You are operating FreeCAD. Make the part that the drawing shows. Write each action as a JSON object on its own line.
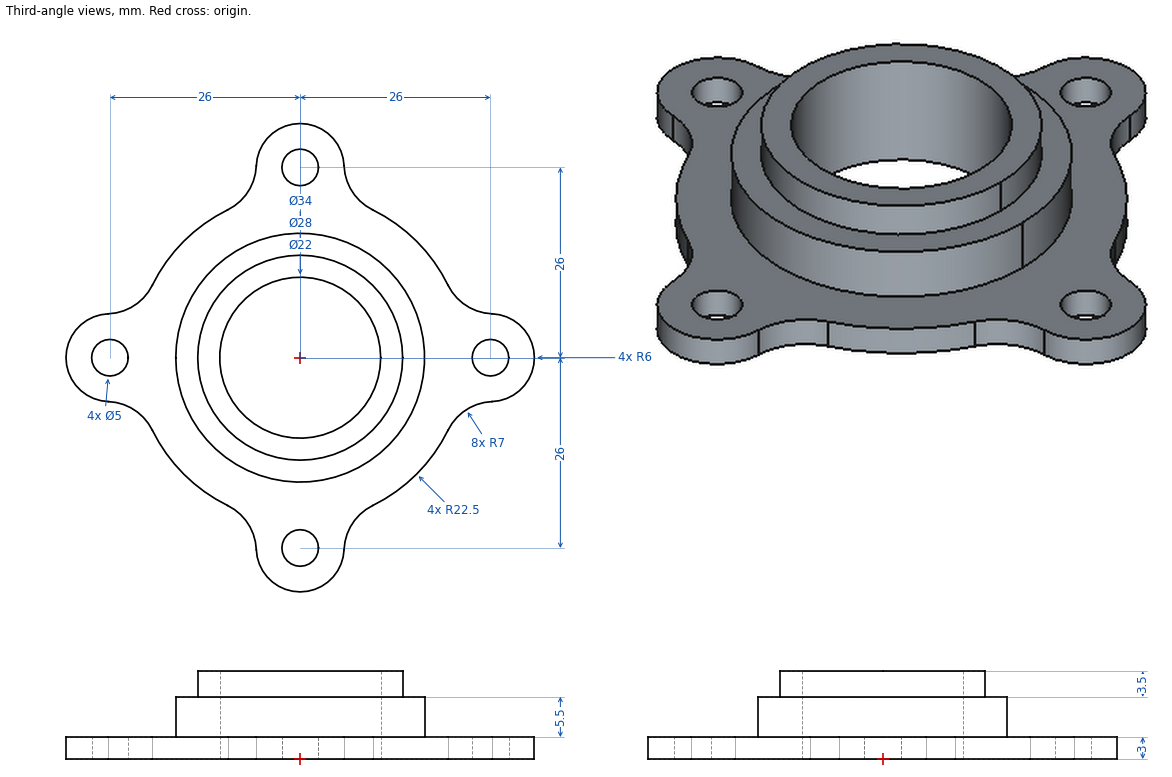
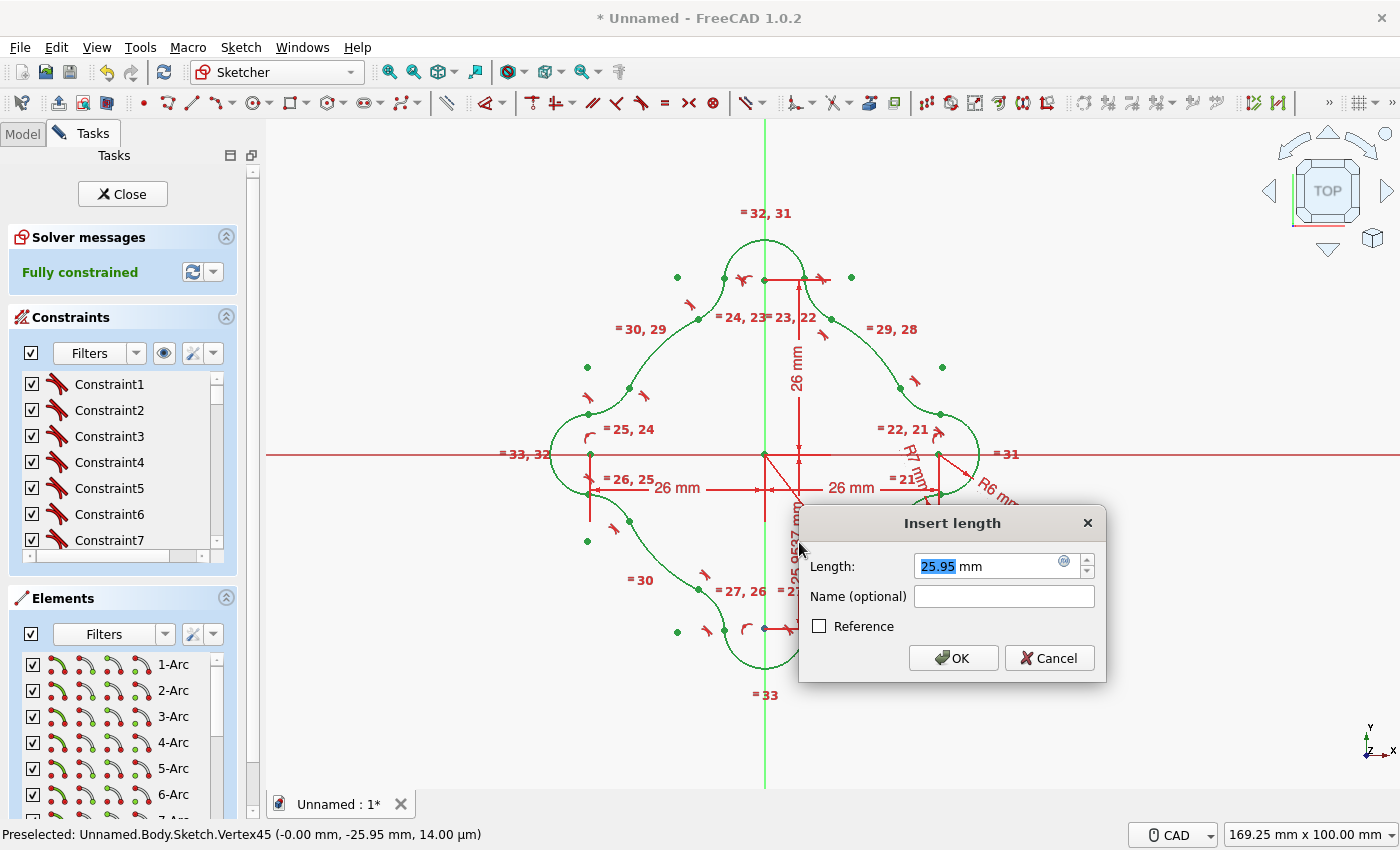
{"action": "type", "text": "26"}
{"action": "key", "text": "Return"}
{"action": "key", "text": "Escape"}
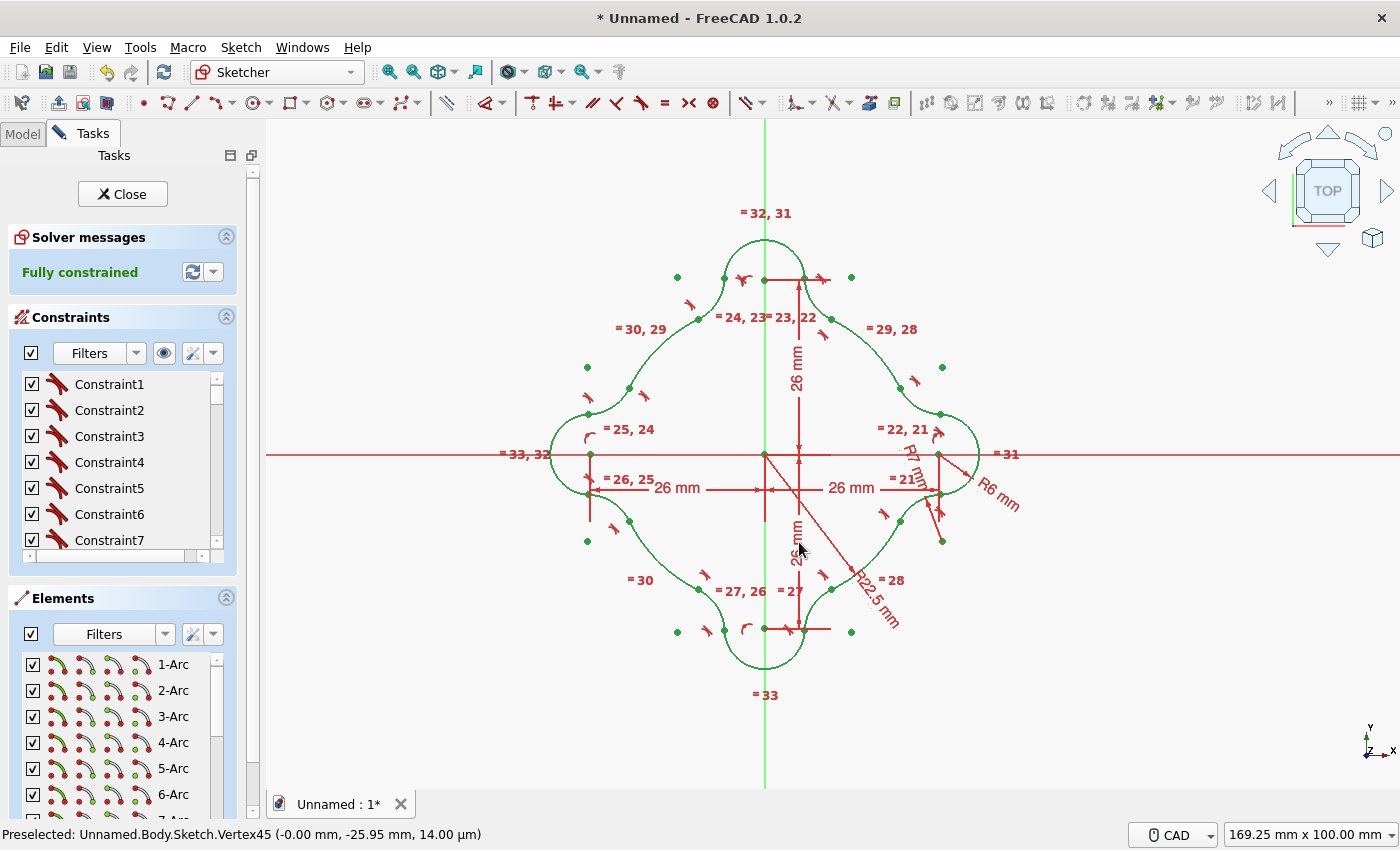
{"action": "left_click", "coordinate": [123, 194]}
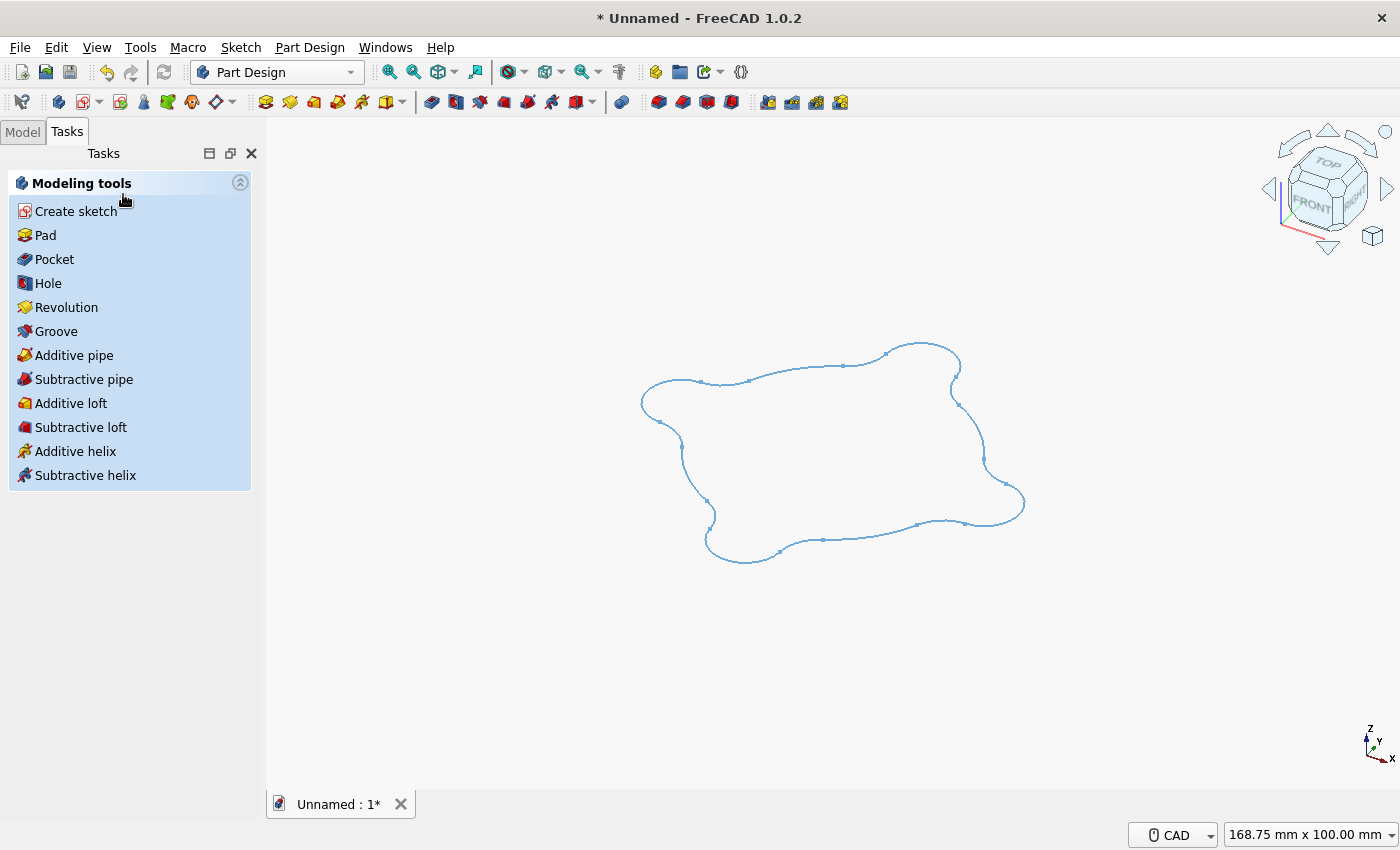
{"action": "left_click", "coordinate": [266, 102]}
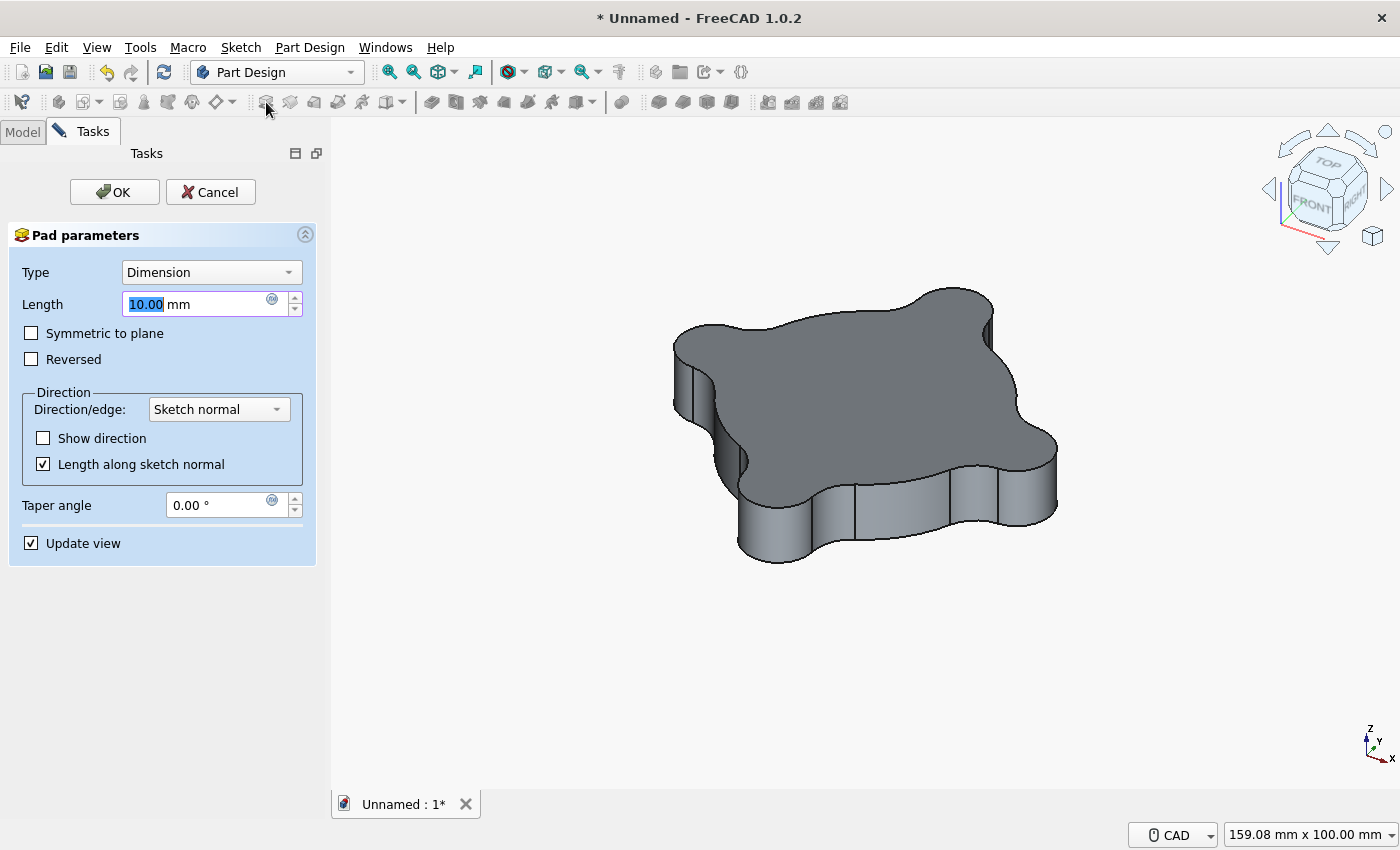
{"action": "type", "text": "3"}
{"action": "key", "text": "Tab"}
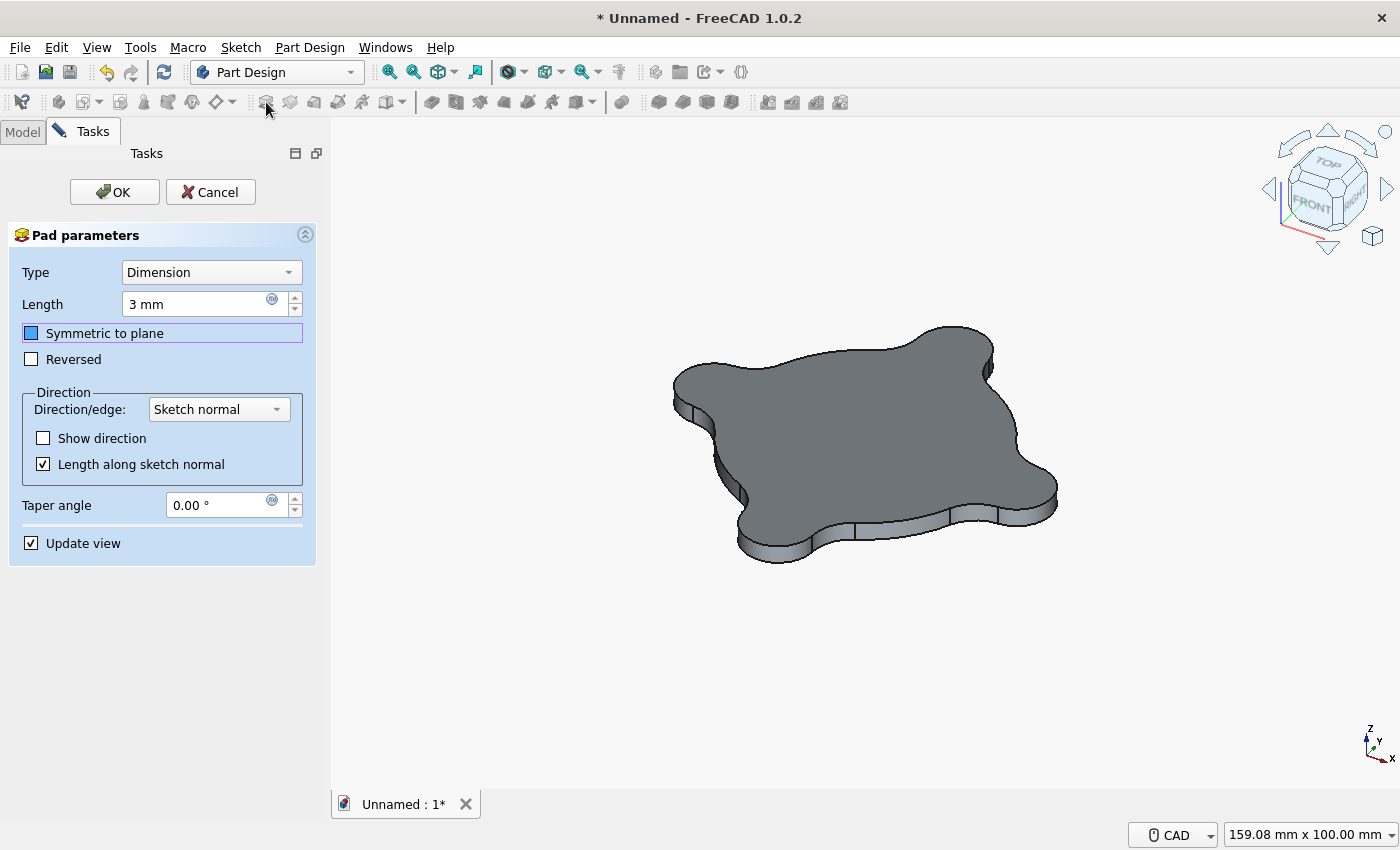
{"action": "left_click", "coordinate": [115, 192]}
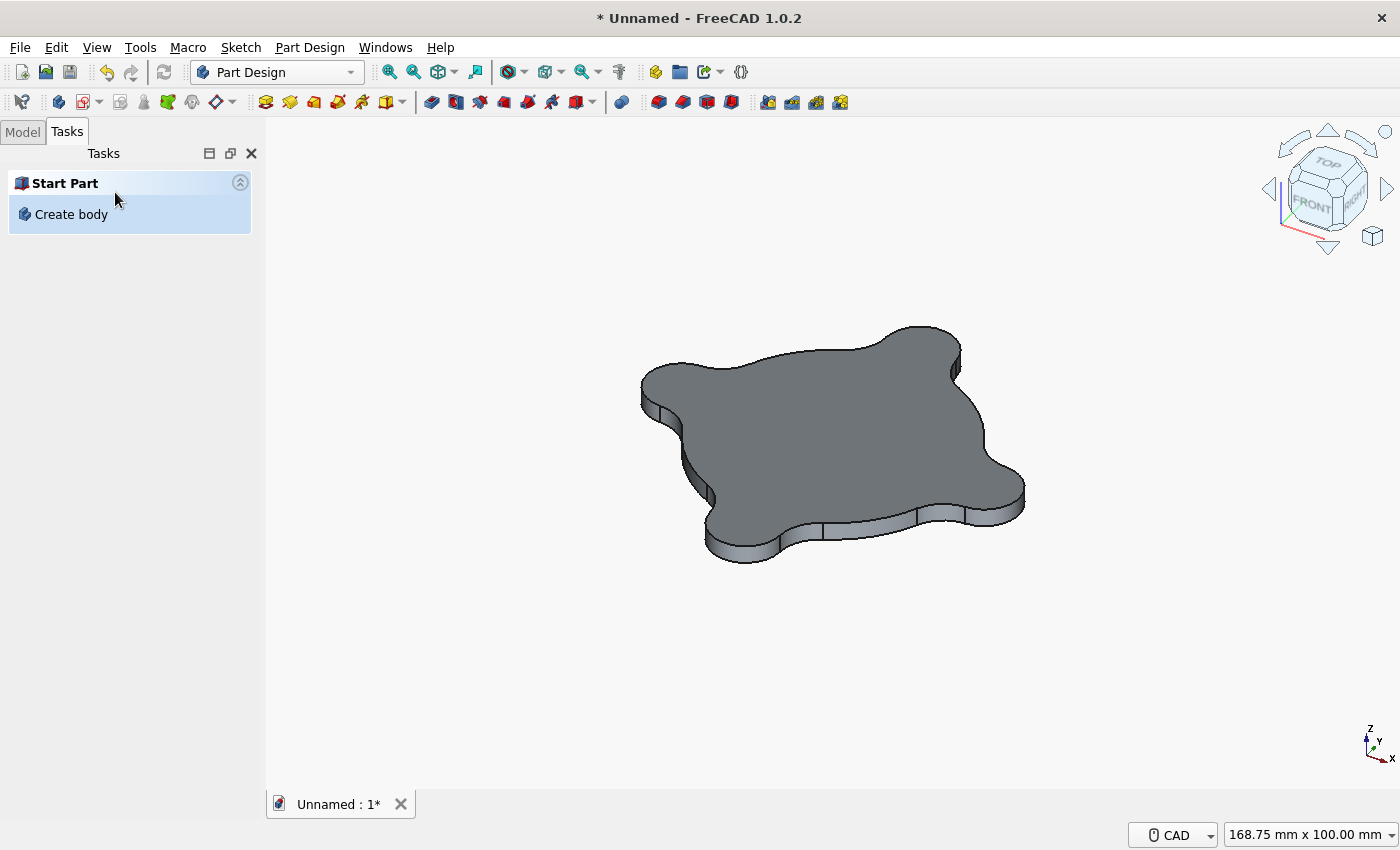
{"action": "left_click", "coordinate": [833, 435]}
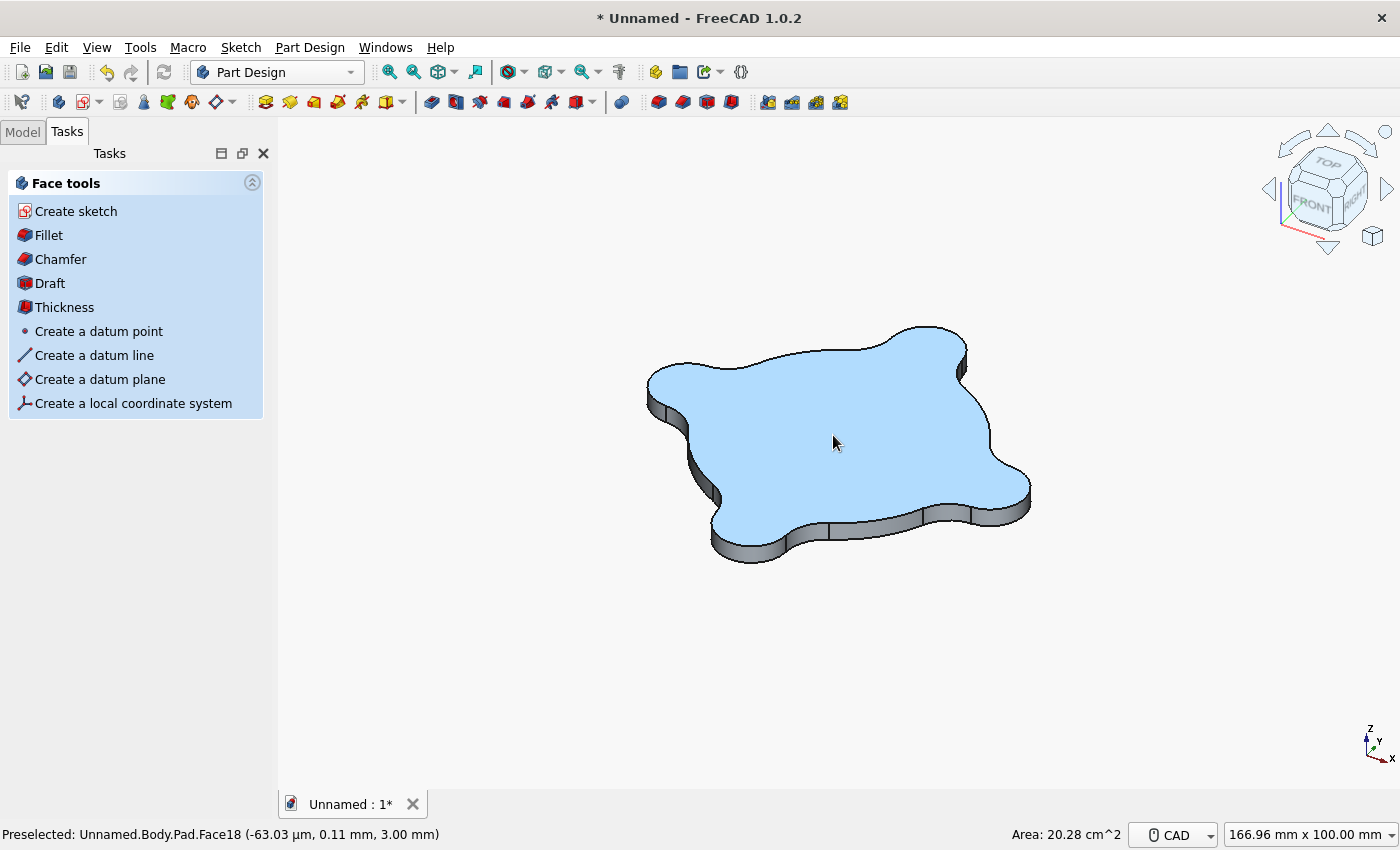
{"action": "left_click", "coordinate": [84, 102]}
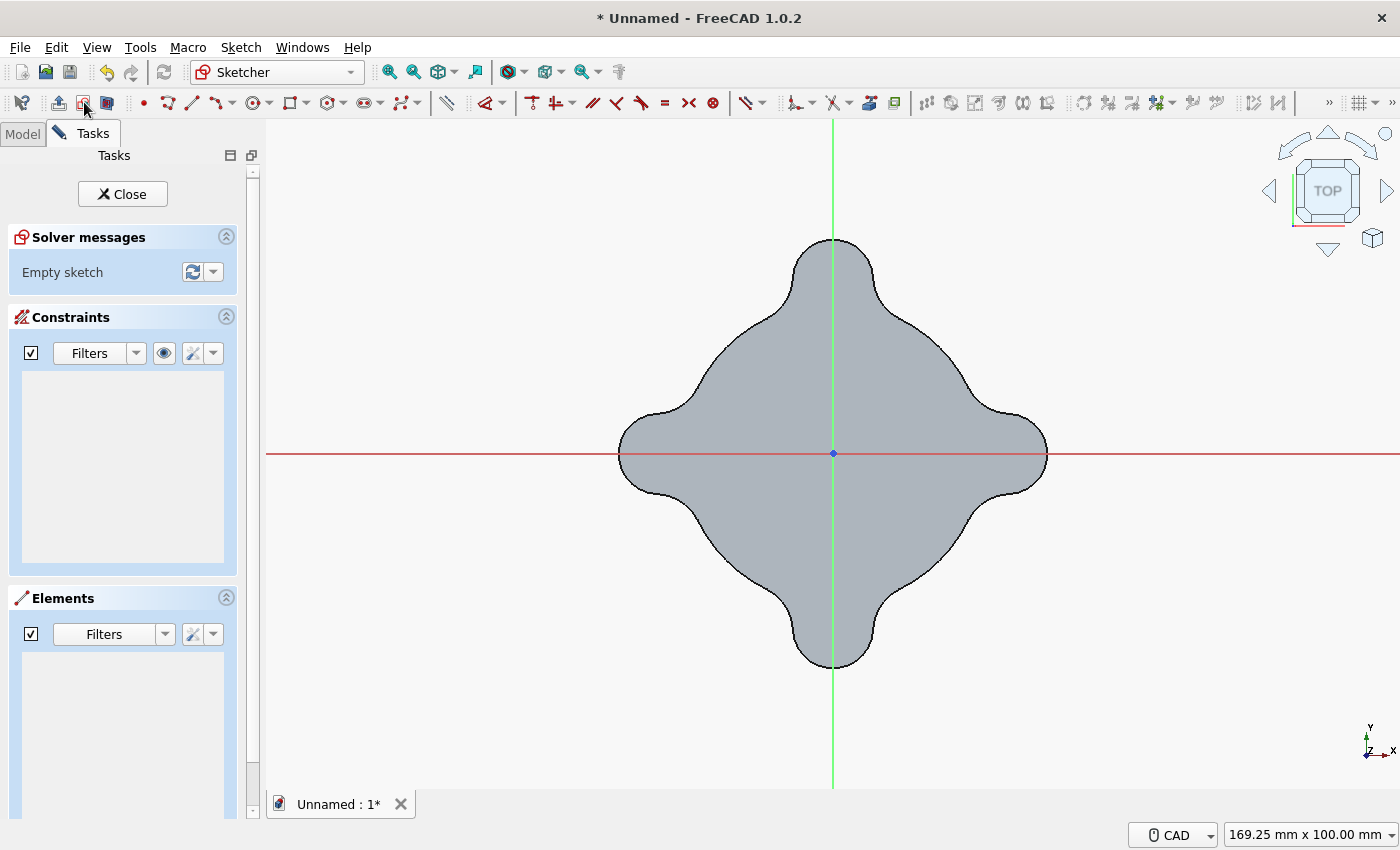
{"action": "scroll", "coordinate": [916, 454], "scroll_direction": "up", "scroll_amount": 3}